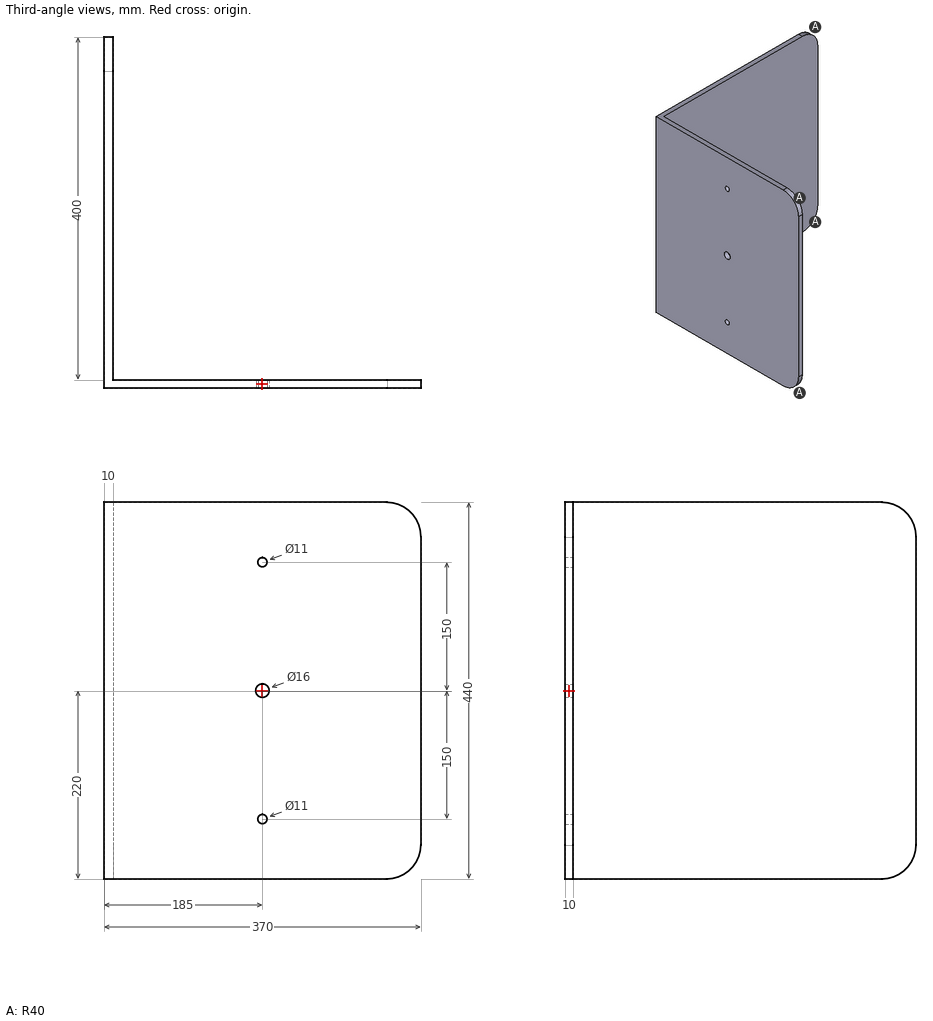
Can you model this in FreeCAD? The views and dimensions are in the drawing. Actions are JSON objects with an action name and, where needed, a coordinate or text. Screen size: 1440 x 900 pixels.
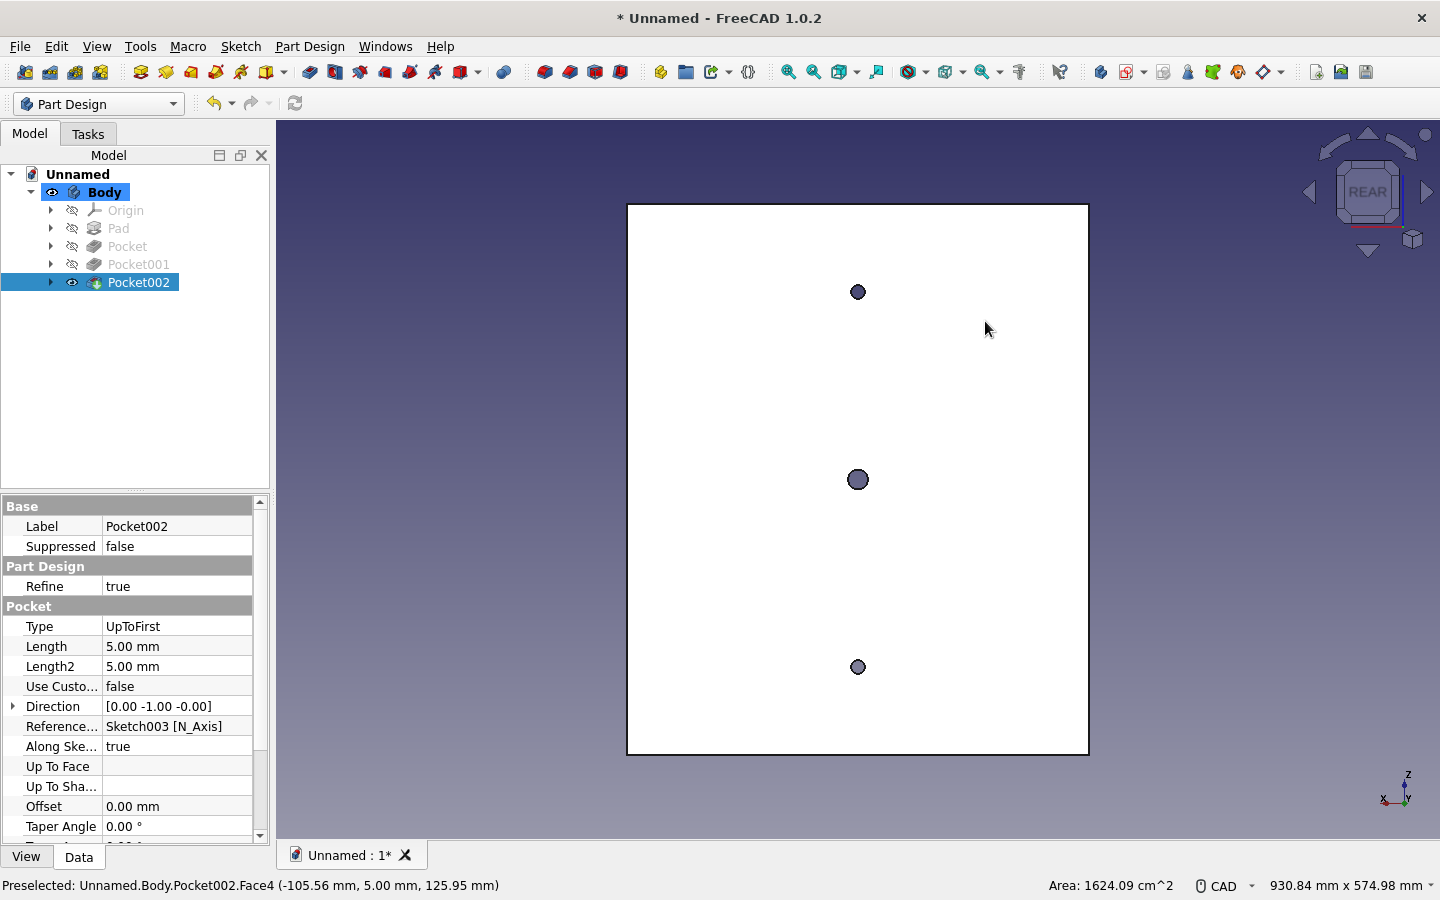
{"action": "left_click", "coordinate": [1126, 72]}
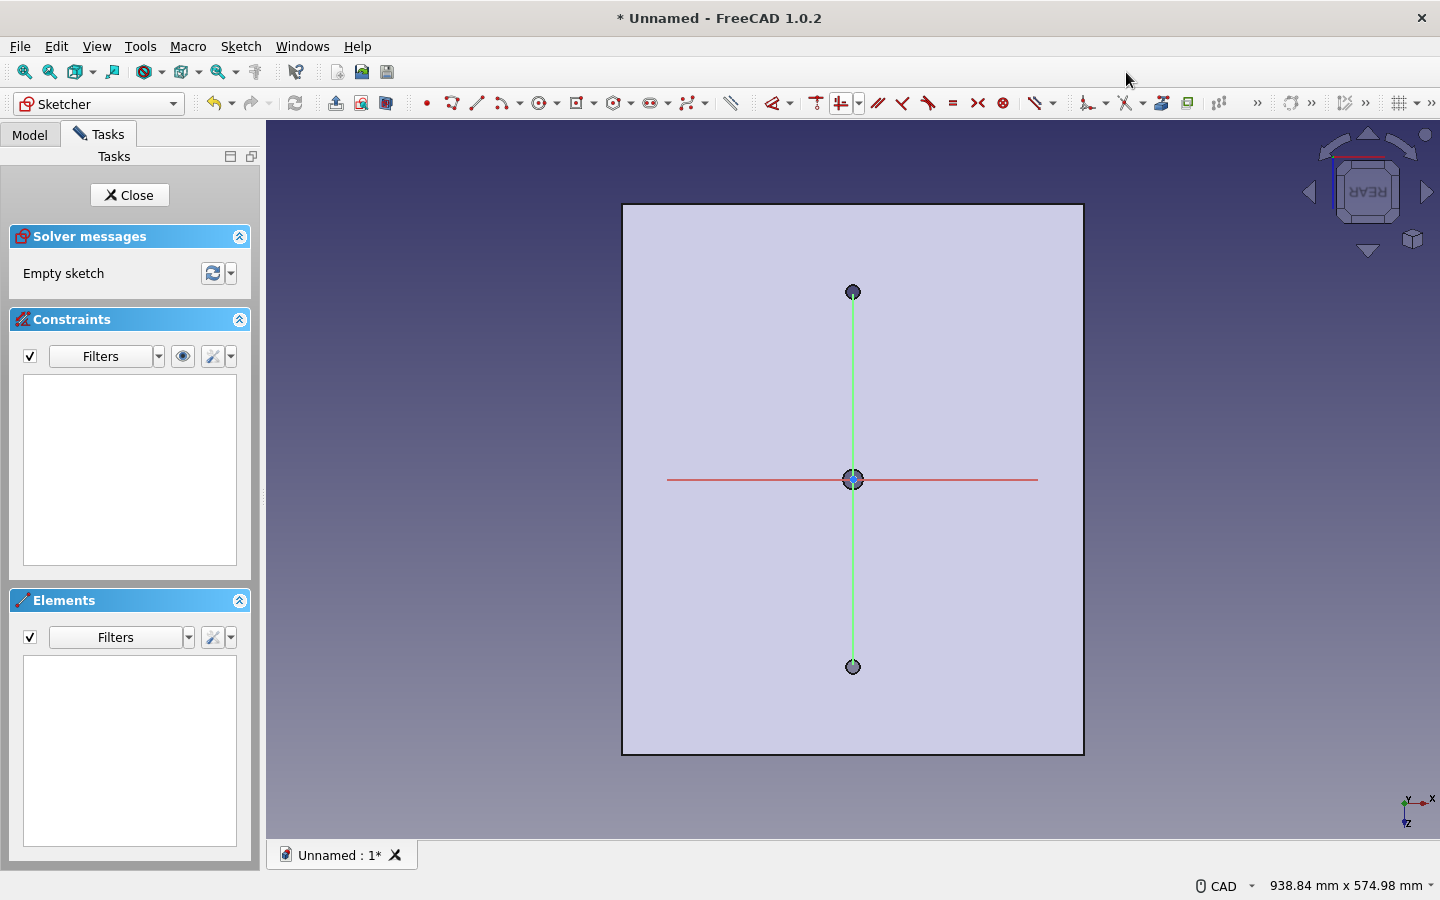
{"action": "key", "text": "g r"}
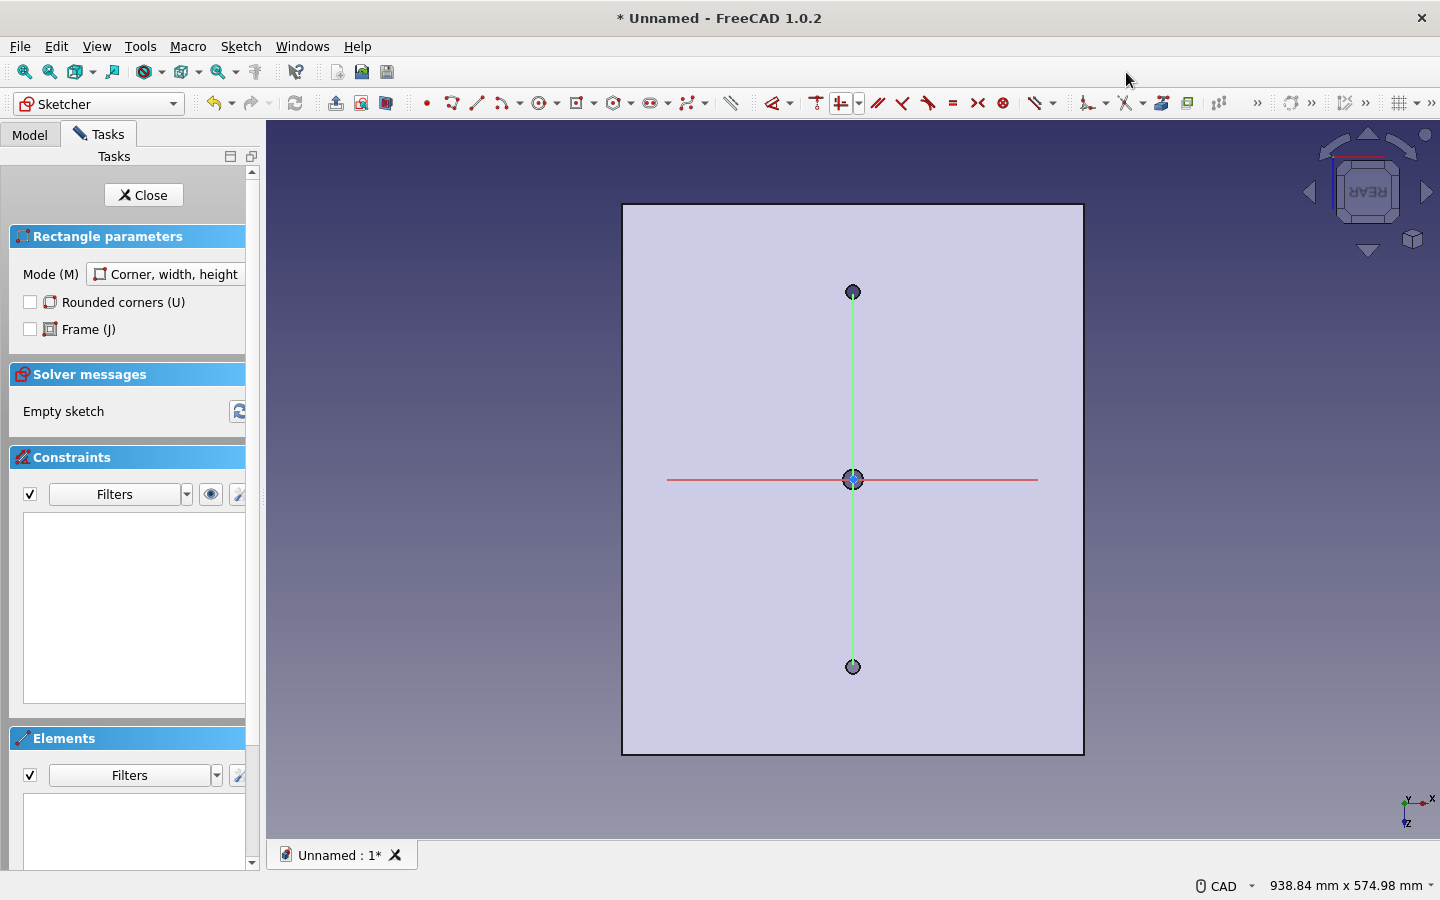
{"action": "scroll", "coordinate": [622, 204], "scroll_direction": "up", "scroll_amount": 2}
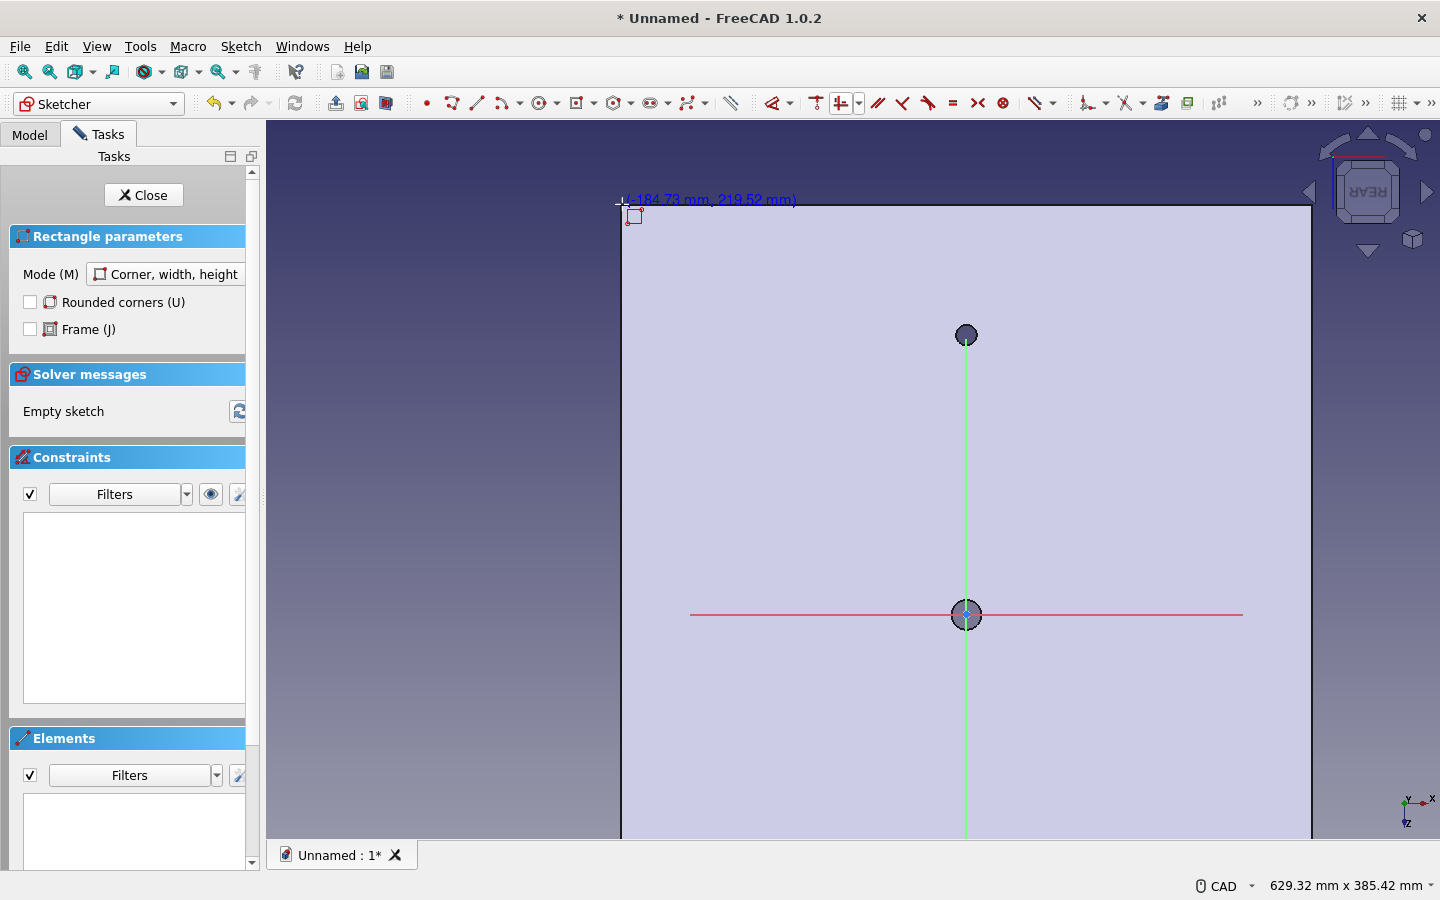
{"action": "left_click", "coordinate": [621, 205]}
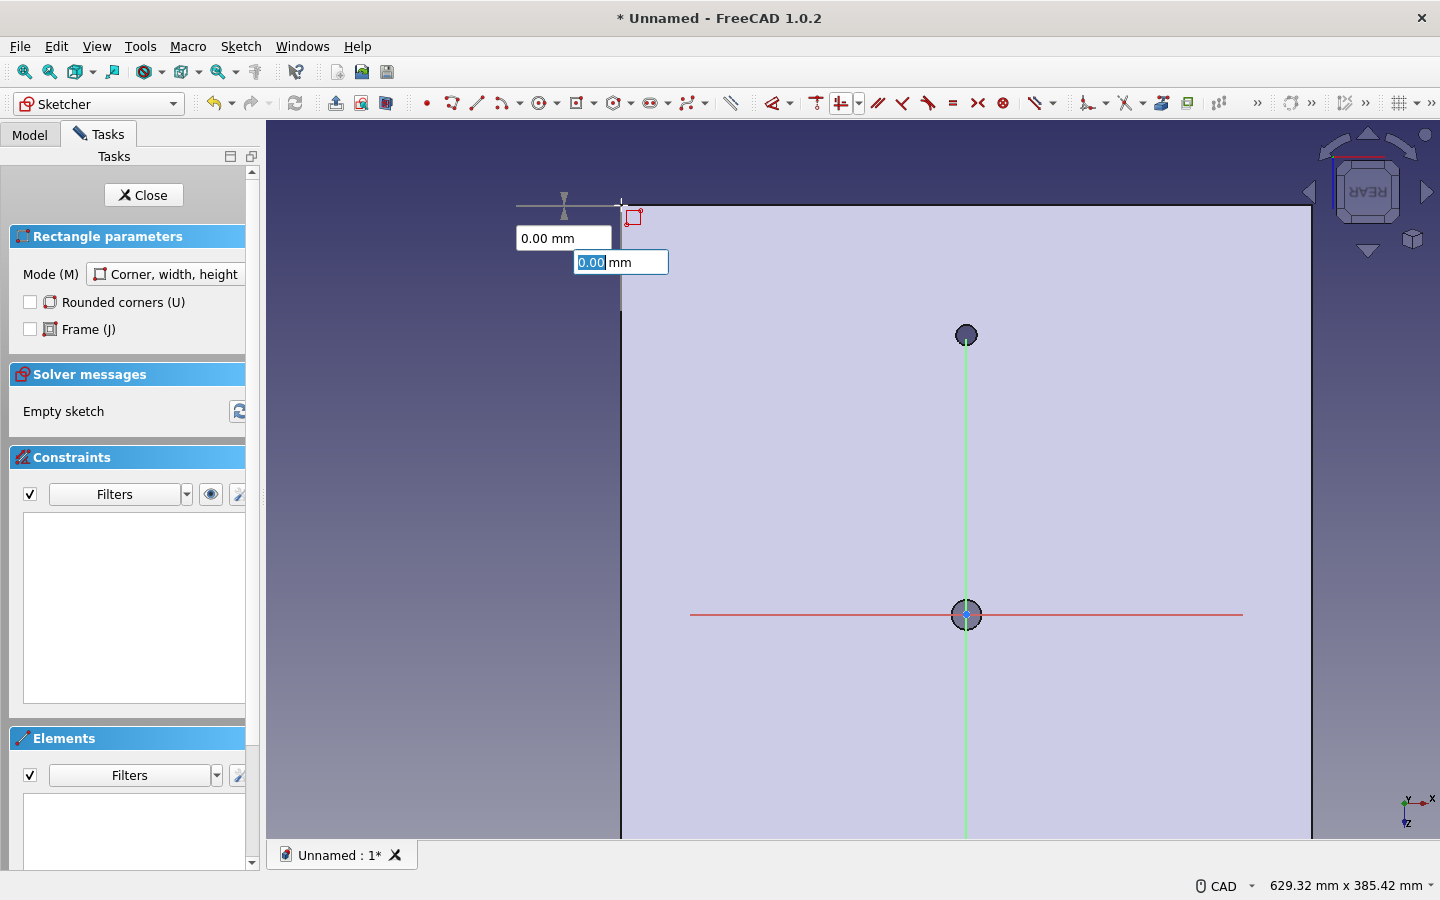
{"action": "scroll", "coordinate": [773, 315], "scroll_direction": "down", "scroll_amount": 3}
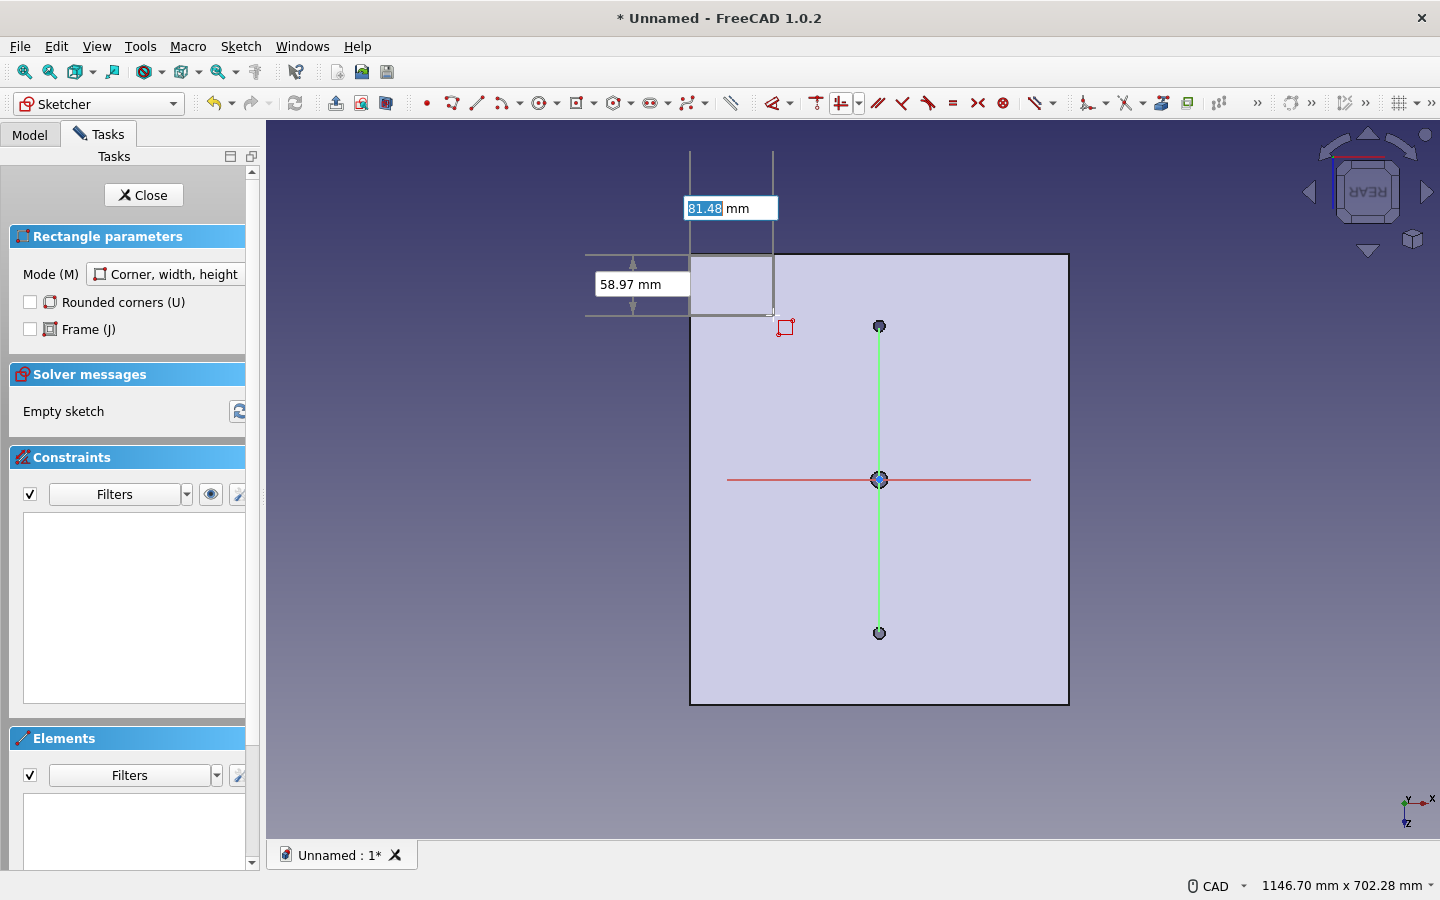
{"action": "left_click", "coordinate": [700, 705]}
{"action": "key", "text": "Escape"}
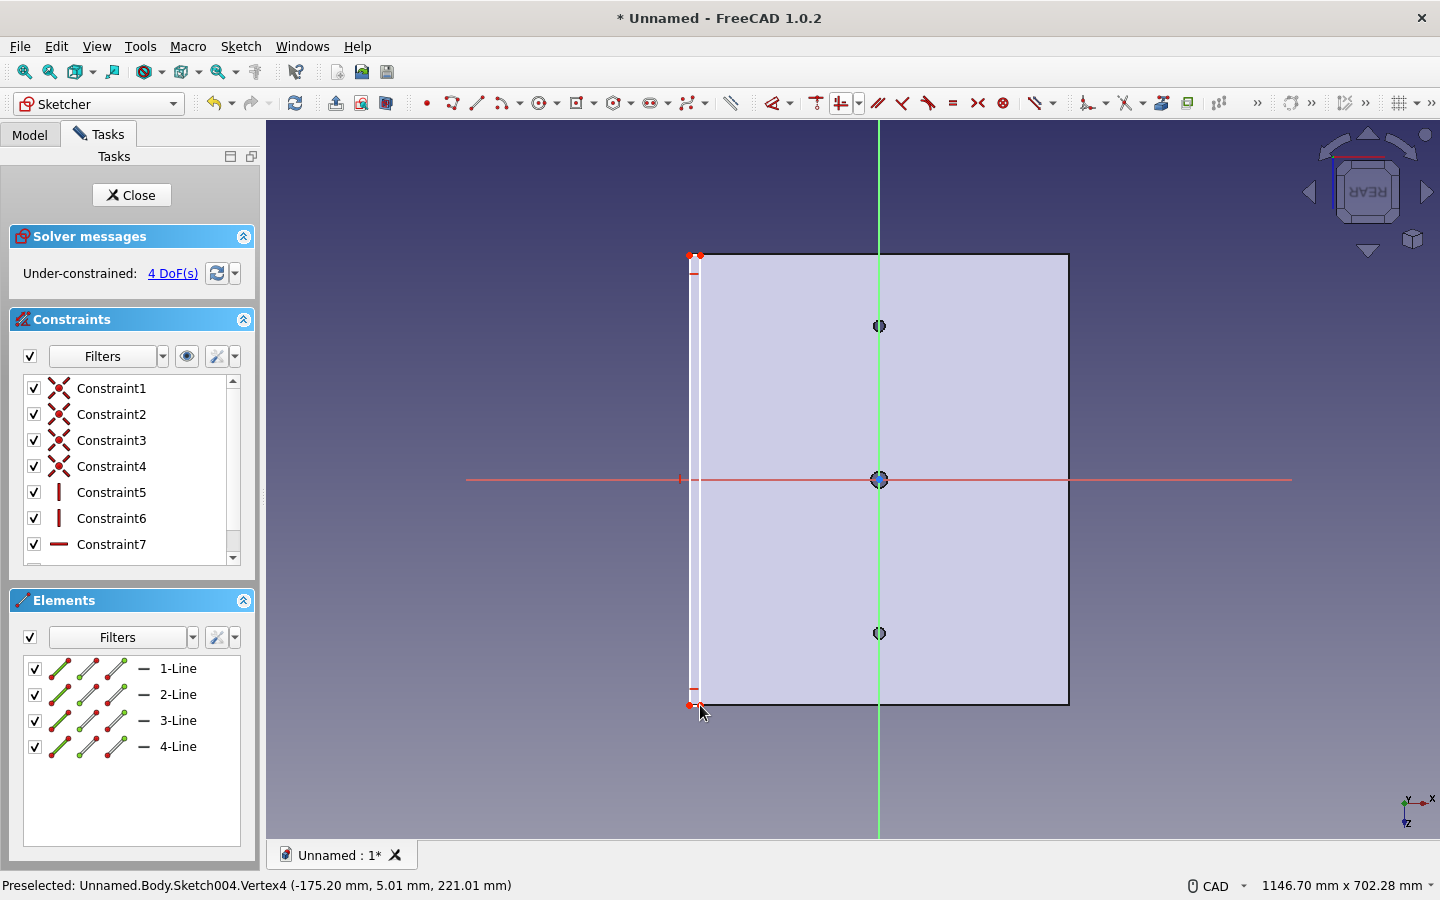
{"action": "left_click", "coordinate": [772, 104]}